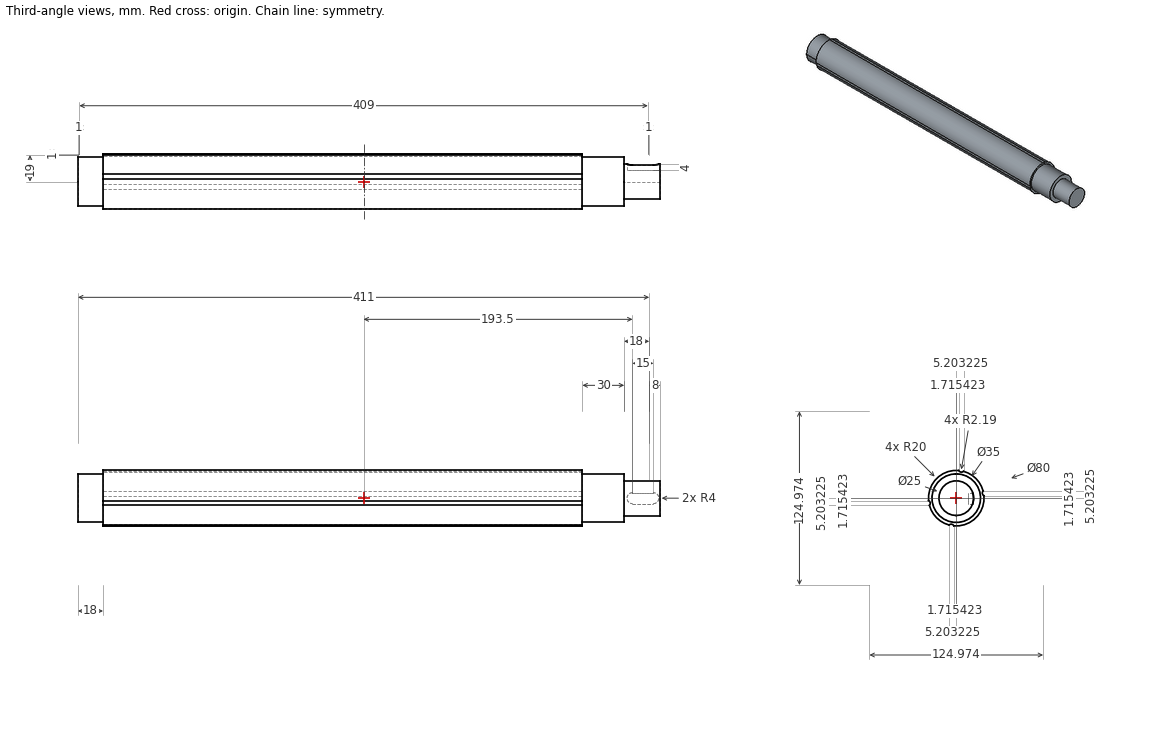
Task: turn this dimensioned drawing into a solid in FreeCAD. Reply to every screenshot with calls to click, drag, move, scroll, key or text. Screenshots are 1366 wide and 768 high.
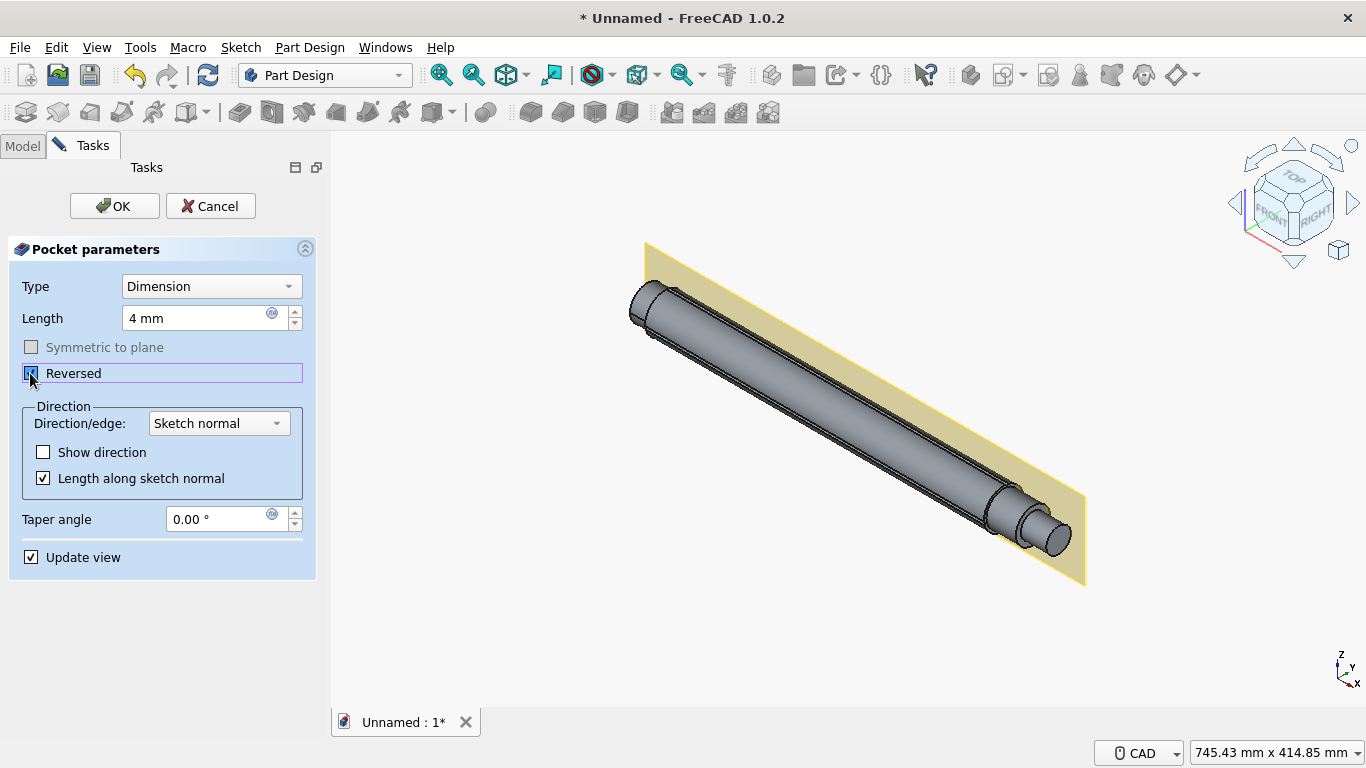
click(115, 206)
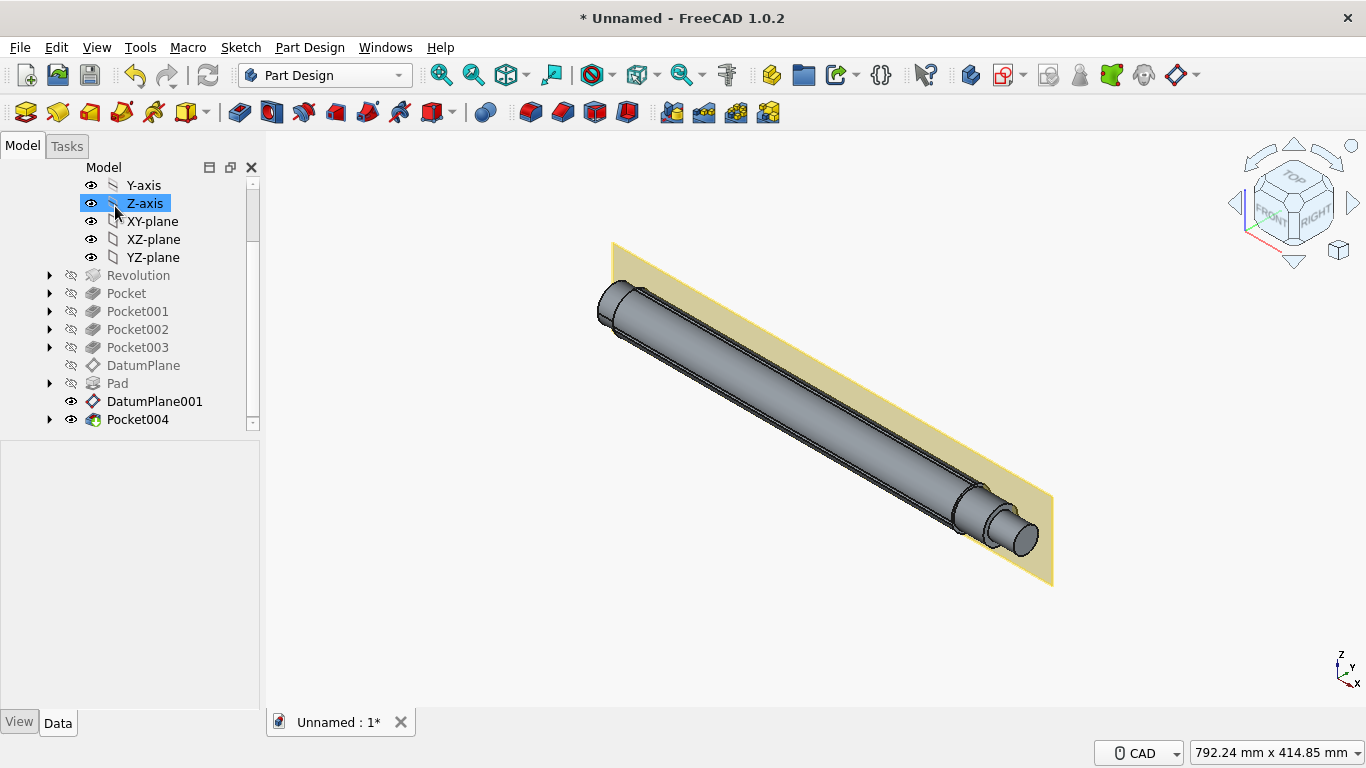
click(116, 401)
key(space)